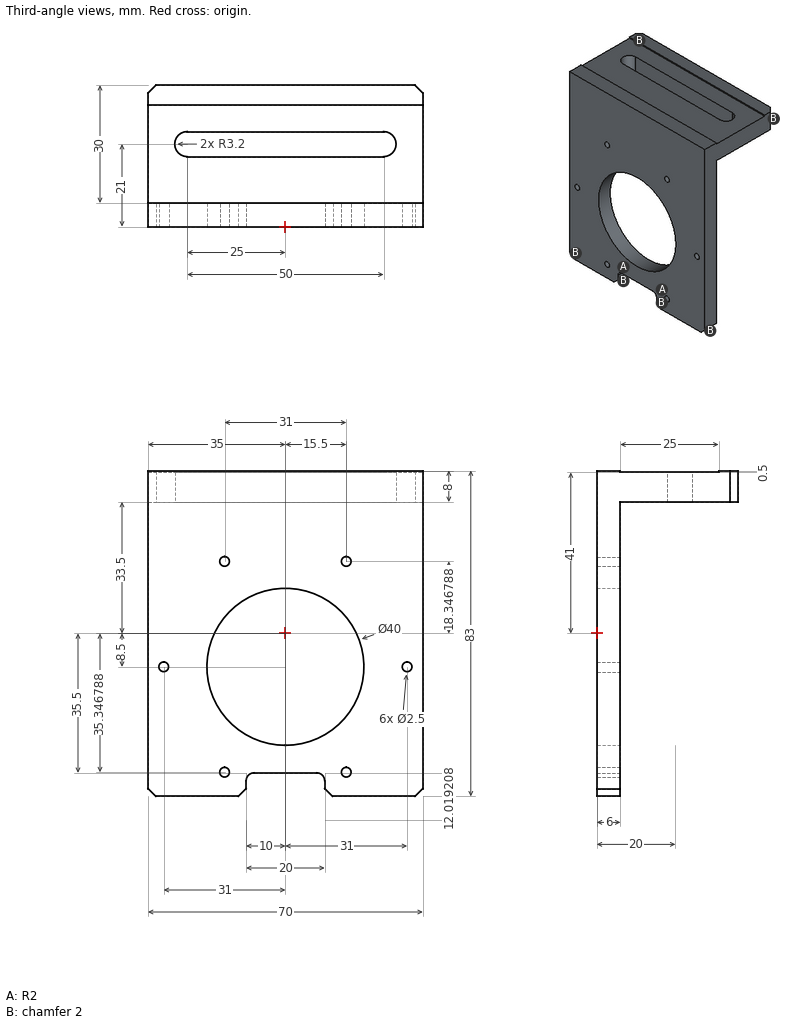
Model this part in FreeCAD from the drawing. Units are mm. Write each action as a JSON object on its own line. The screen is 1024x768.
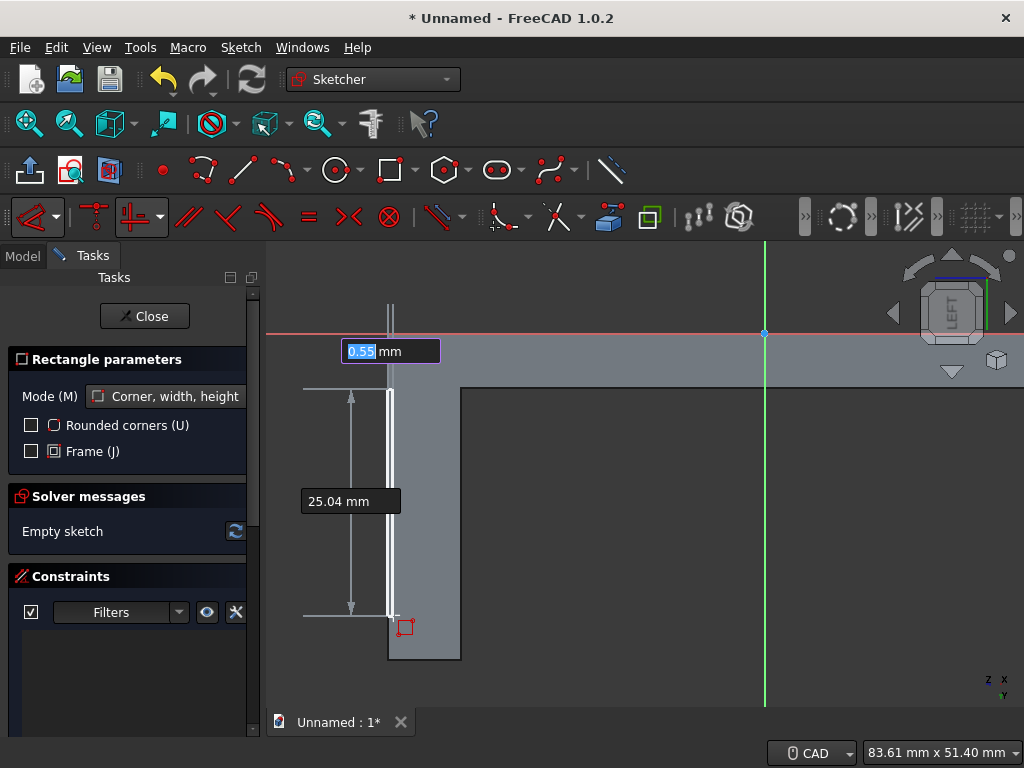
{"action": "type", "text": "0.5"}
{"action": "key", "text": "Tab"}
{"action": "type", "text": "25"}
{"action": "key", "text": "Return"}
{"action": "key", "text": "Escape"}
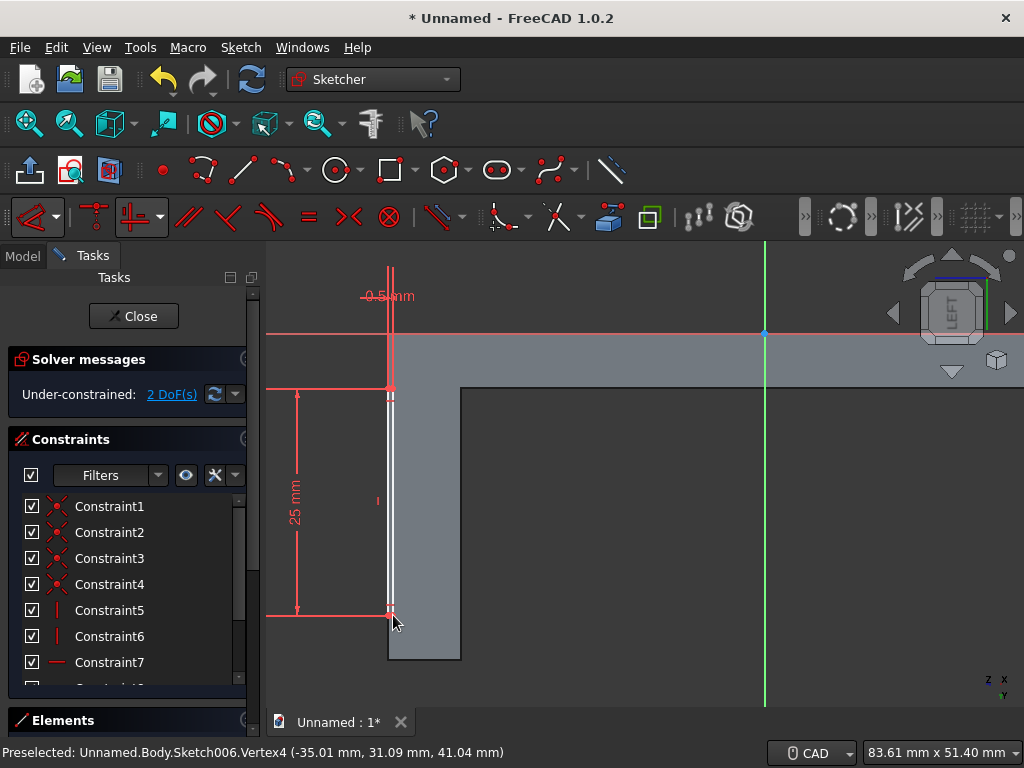
{"action": "scroll", "coordinate": [388, 389], "scroll_direction": "up", "scroll_amount": 5}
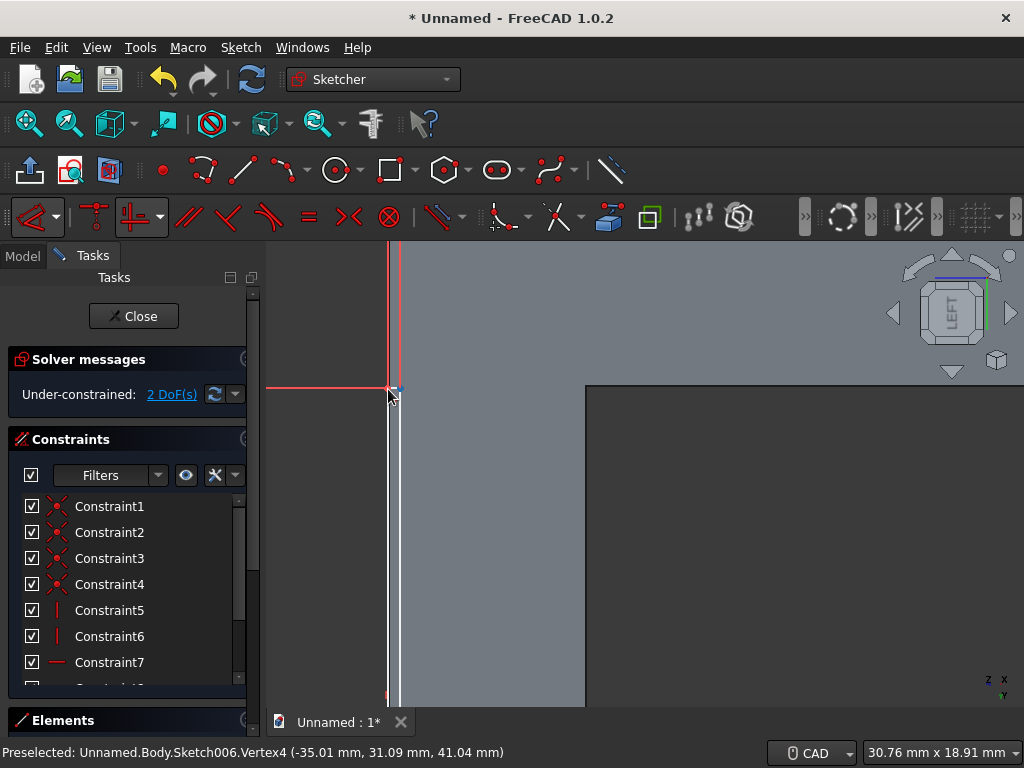
{"action": "left_click", "coordinate": [388, 388]}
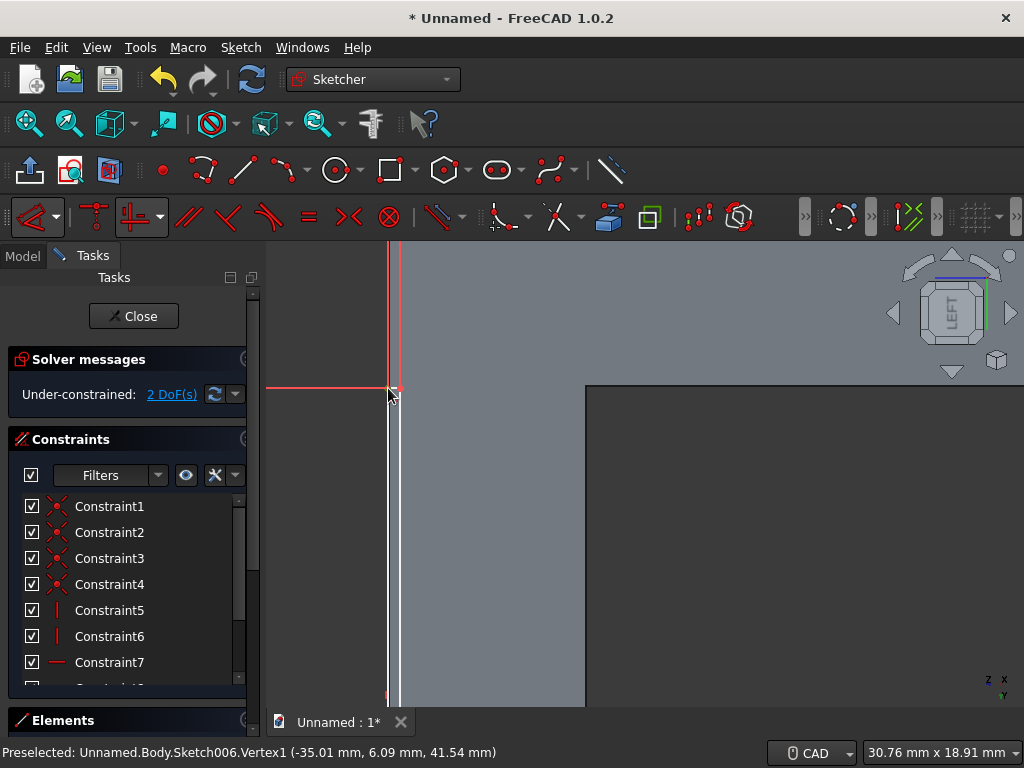
{"action": "left_click", "coordinate": [58, 218]}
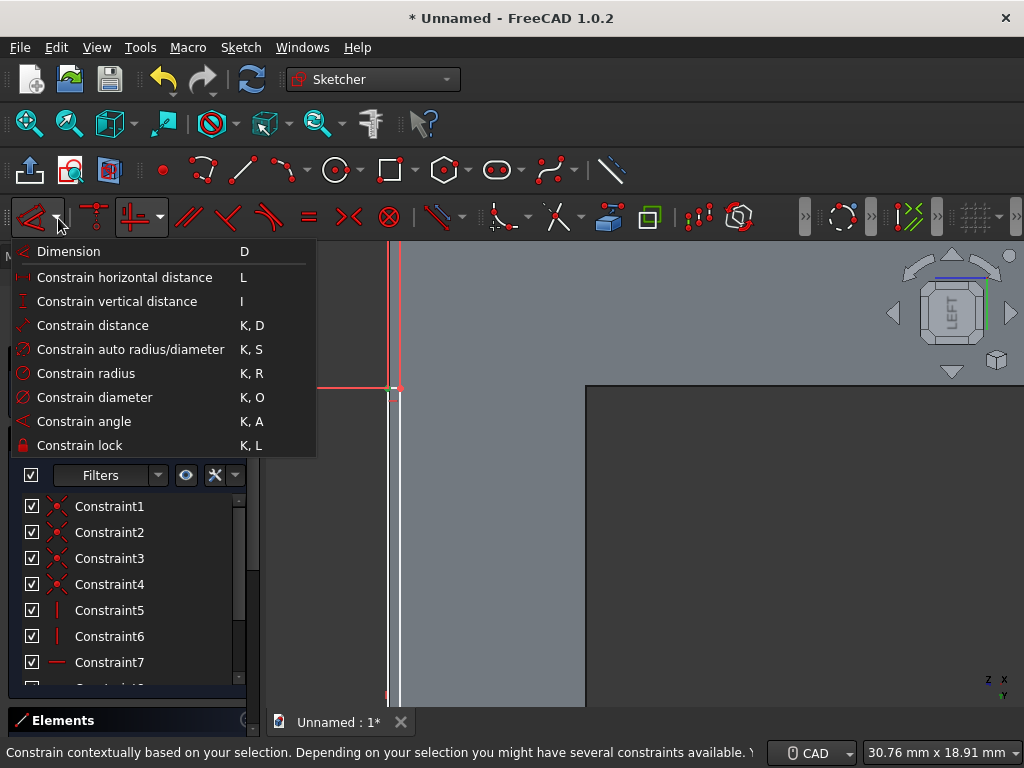
{"action": "left_click", "coordinate": [164, 301]}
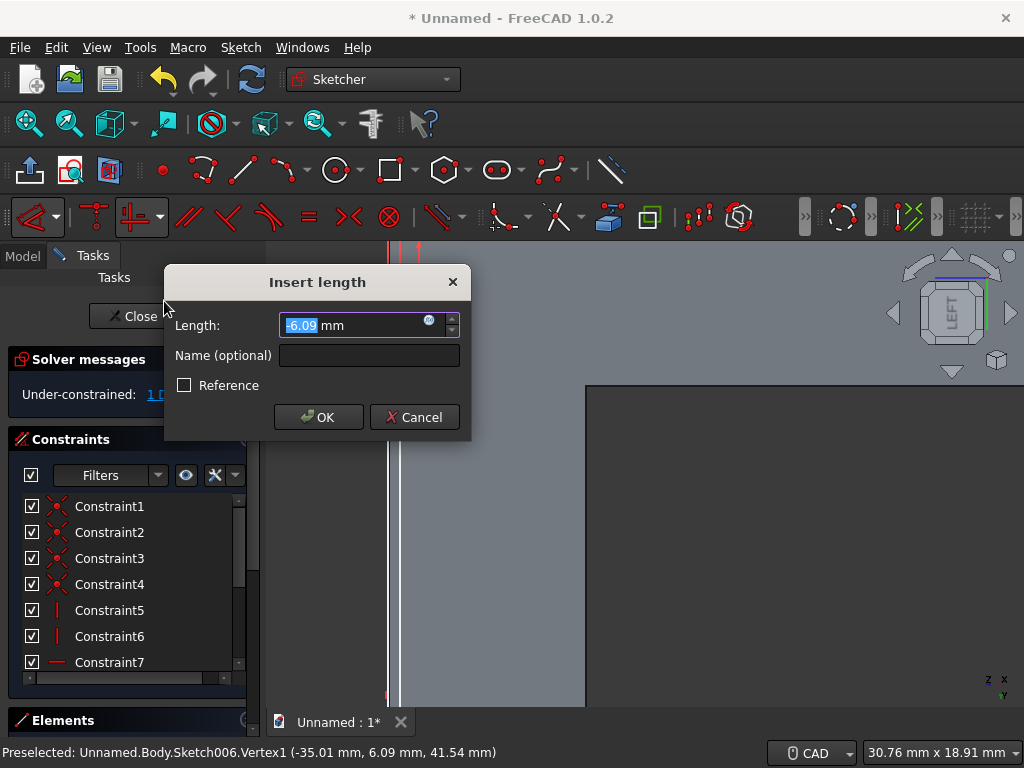
{"action": "type", "text": "-6"}
{"action": "key", "text": "Return"}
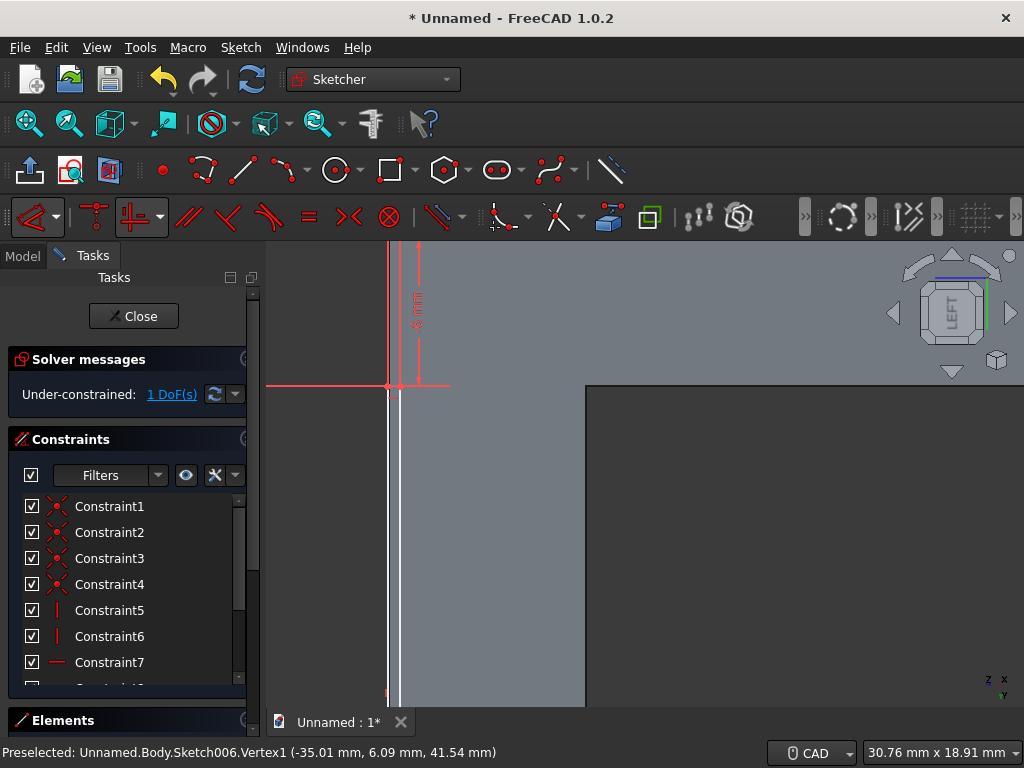
{"action": "scroll", "coordinate": [388, 389], "scroll_direction": "down", "scroll_amount": 5}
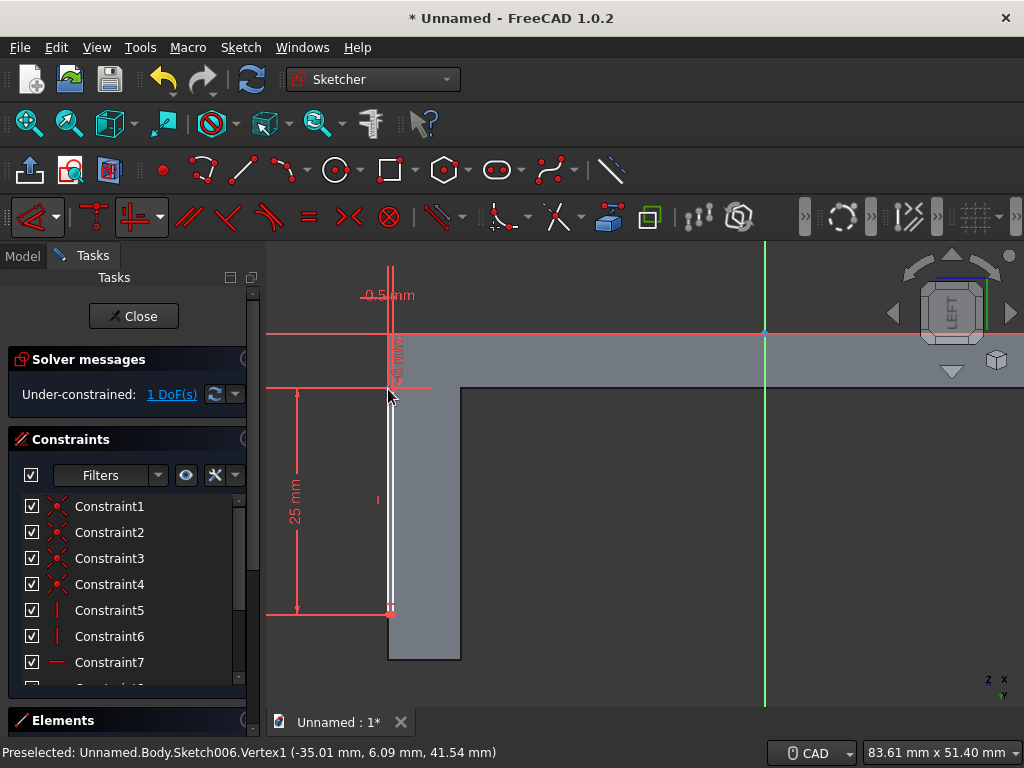
{"action": "scroll", "coordinate": [393, 615], "scroll_direction": "up", "scroll_amount": 5}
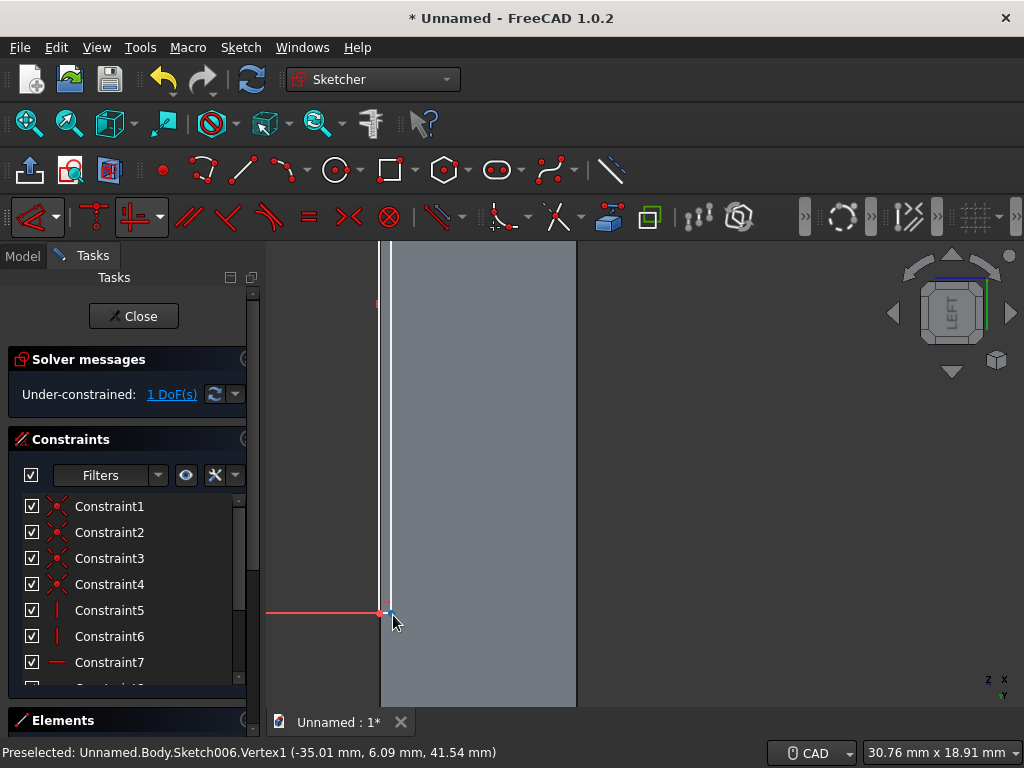
{"action": "left_click", "coordinate": [391, 613]}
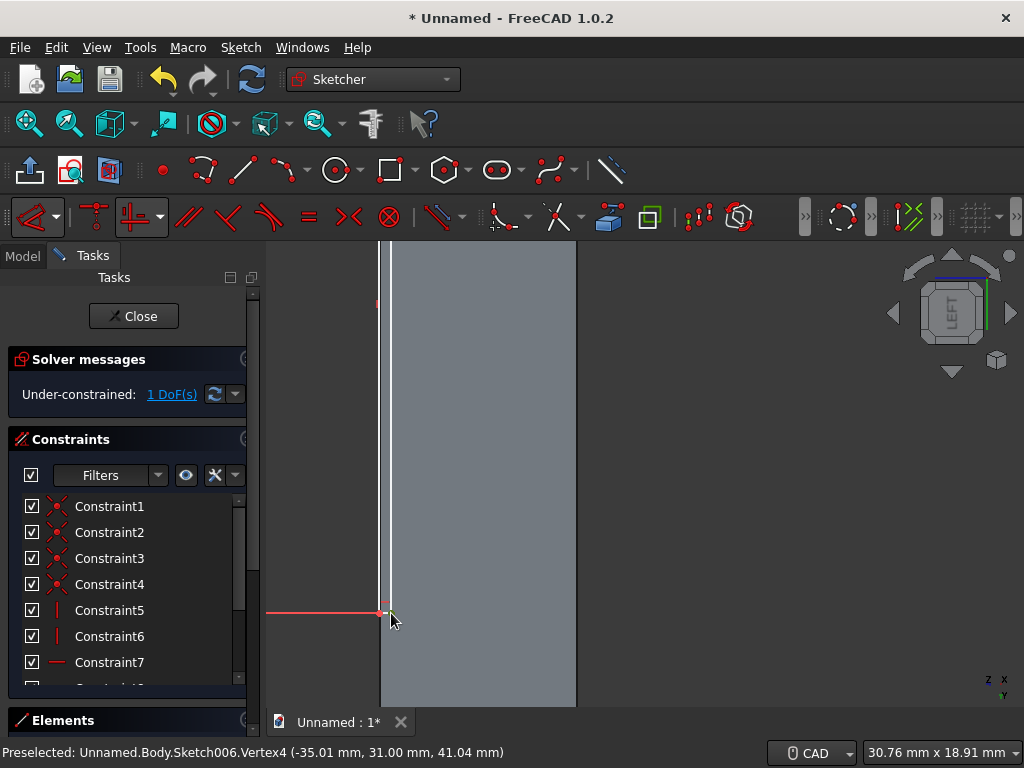
{"action": "left_click", "coordinate": [58, 218]}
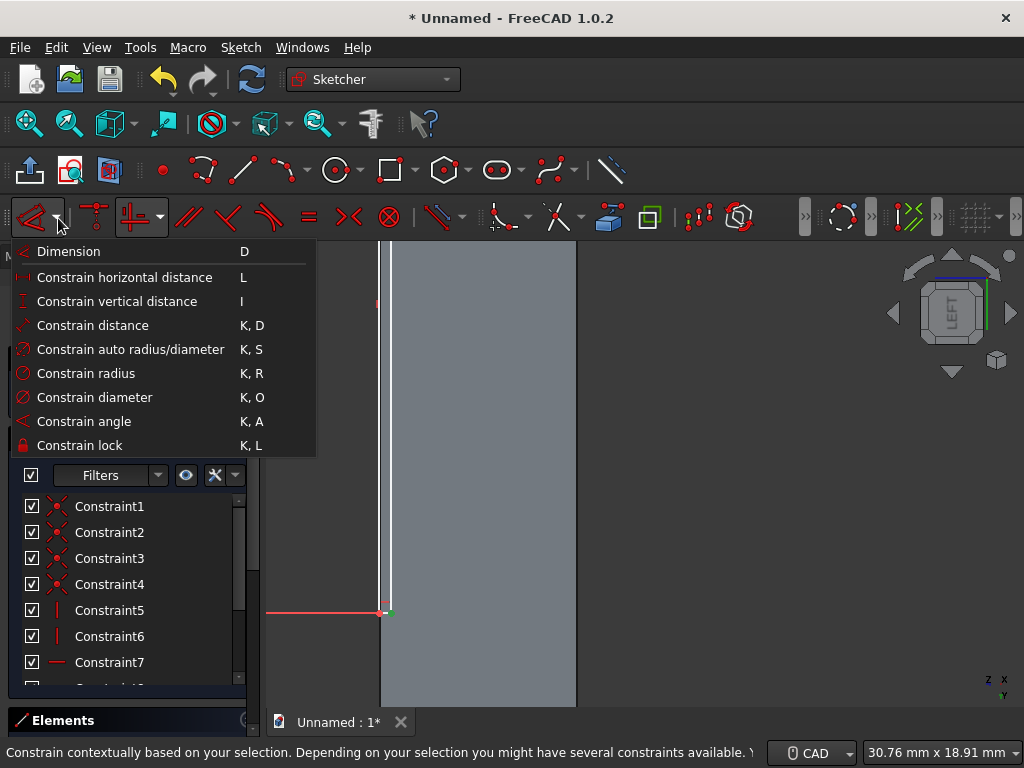
{"action": "left_click", "coordinate": [164, 277]}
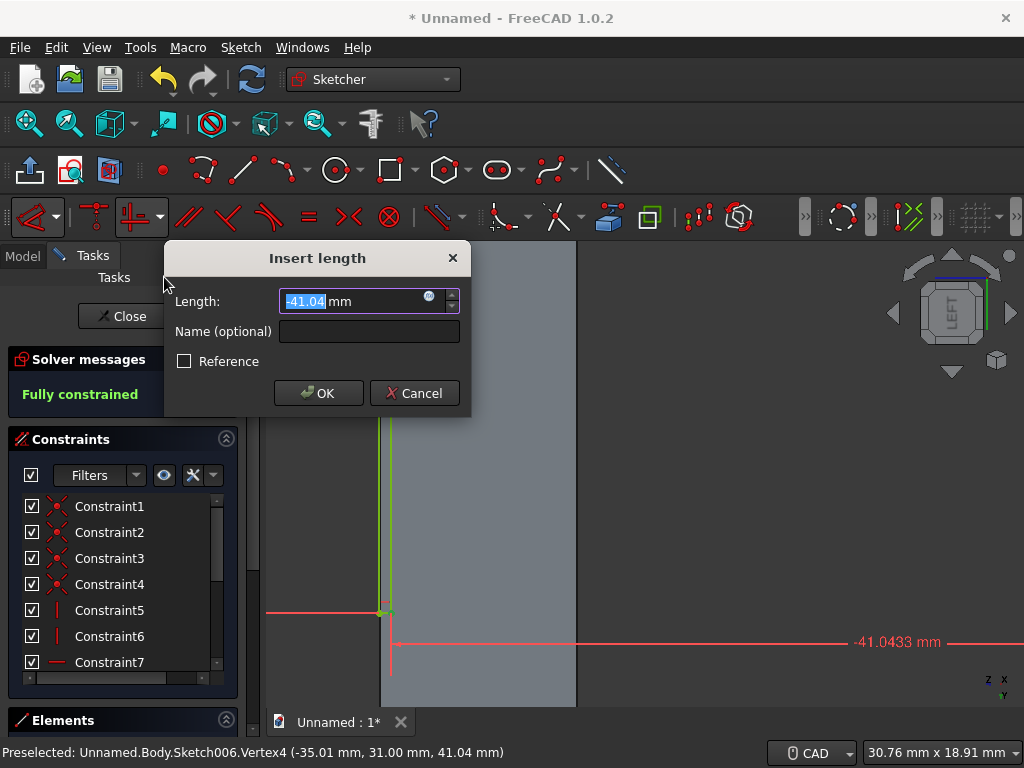
{"action": "type", "text": "-41"}
{"action": "key", "text": "Return"}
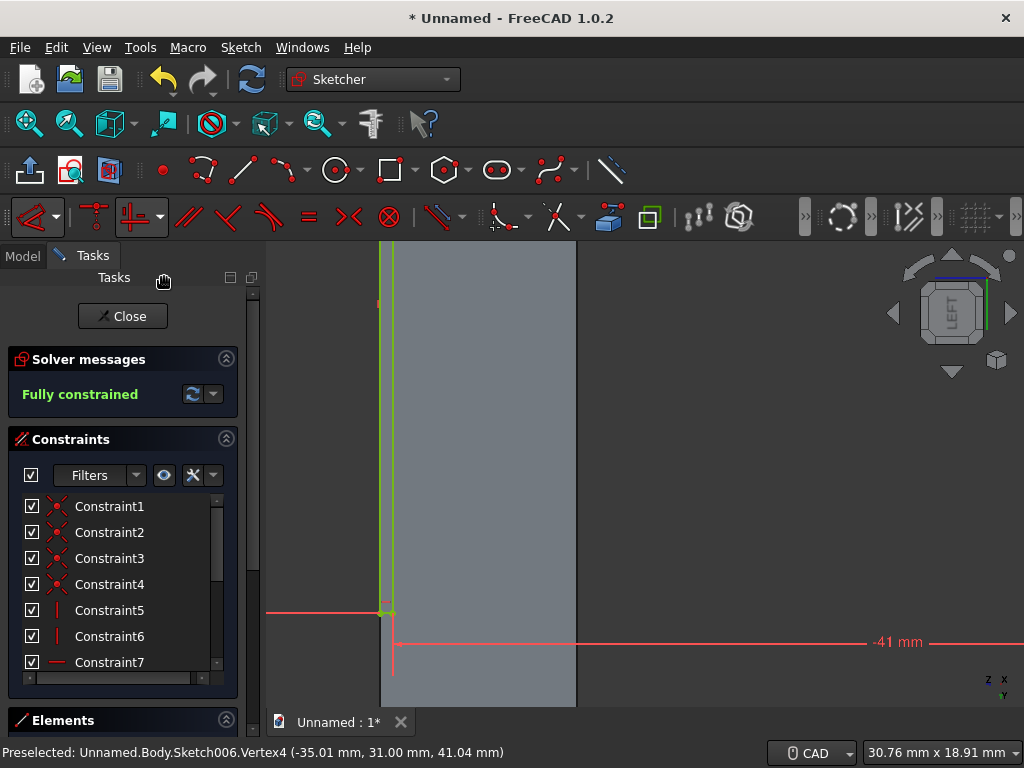
{"action": "left_click", "coordinate": [123, 316]}